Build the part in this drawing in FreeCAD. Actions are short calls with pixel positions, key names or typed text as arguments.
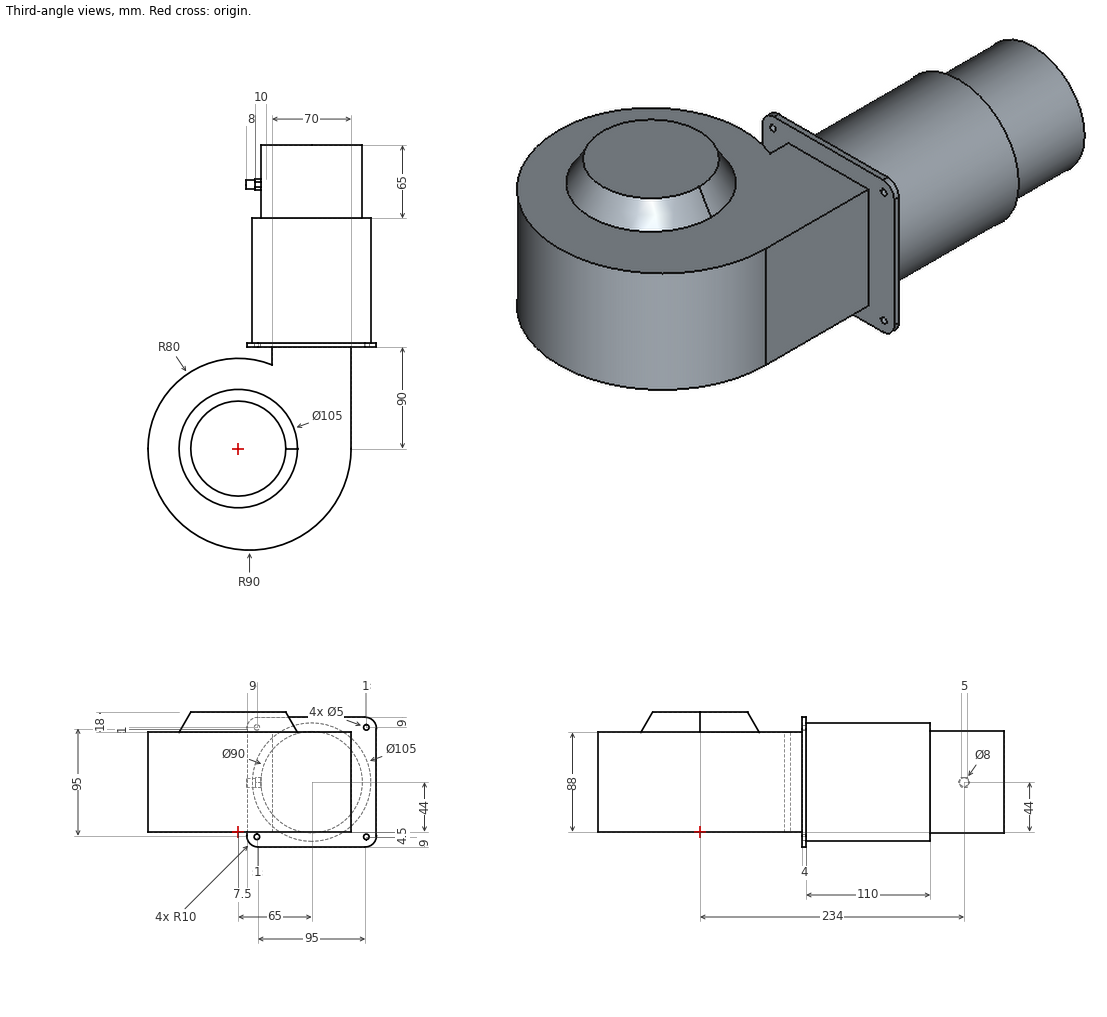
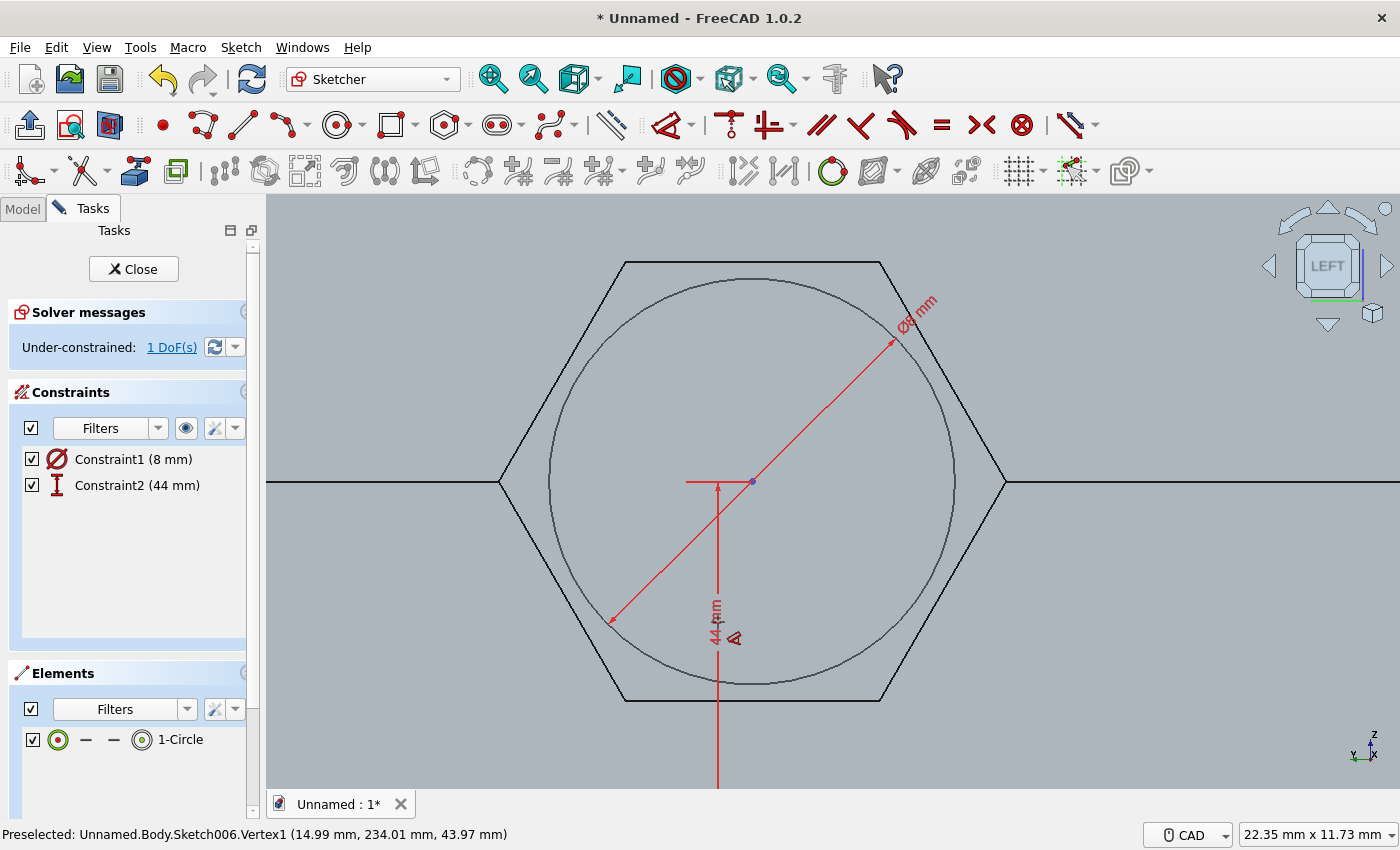
click(752, 482)
click(994, 448)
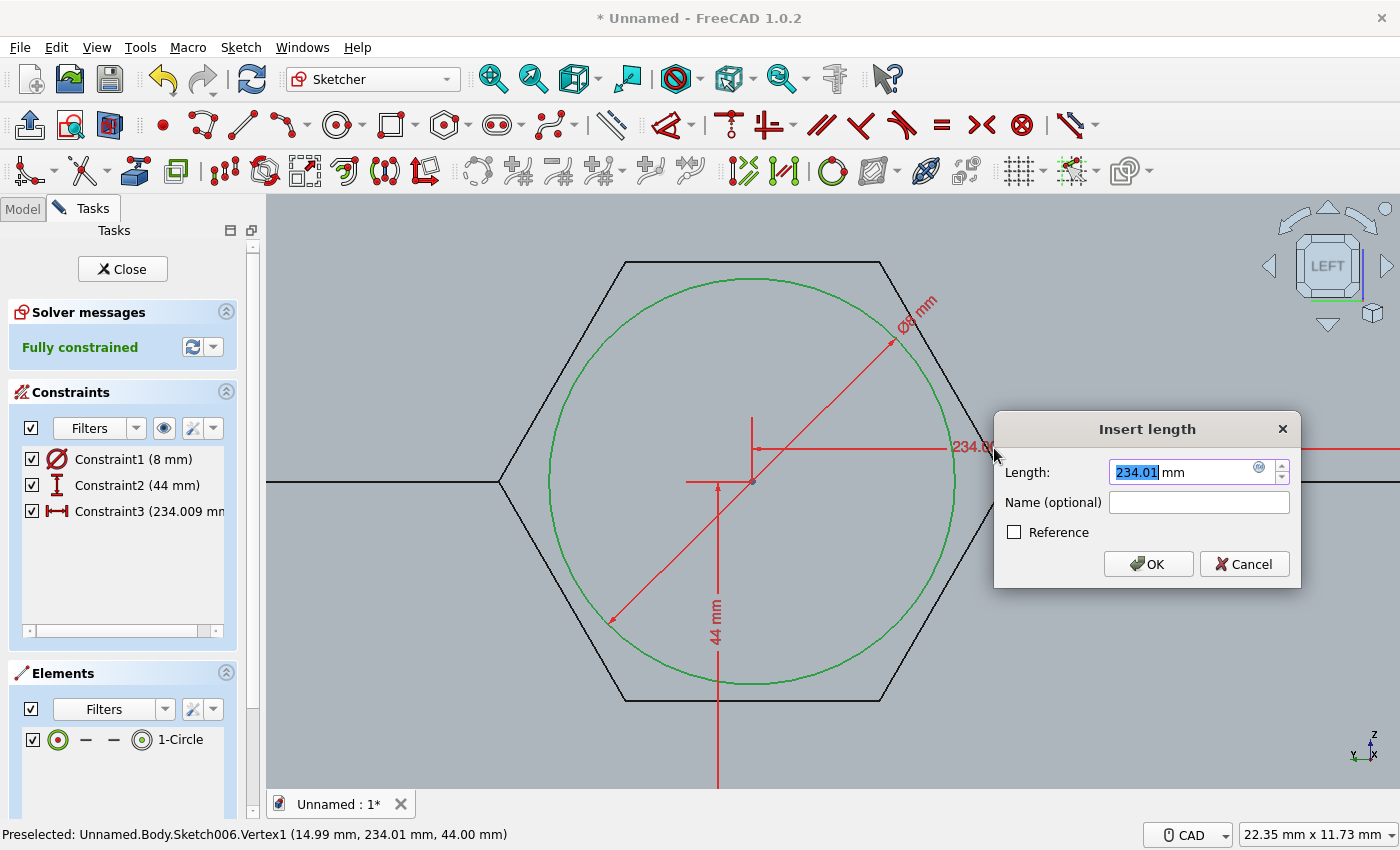
text(234)
key(Return)
key(Escape)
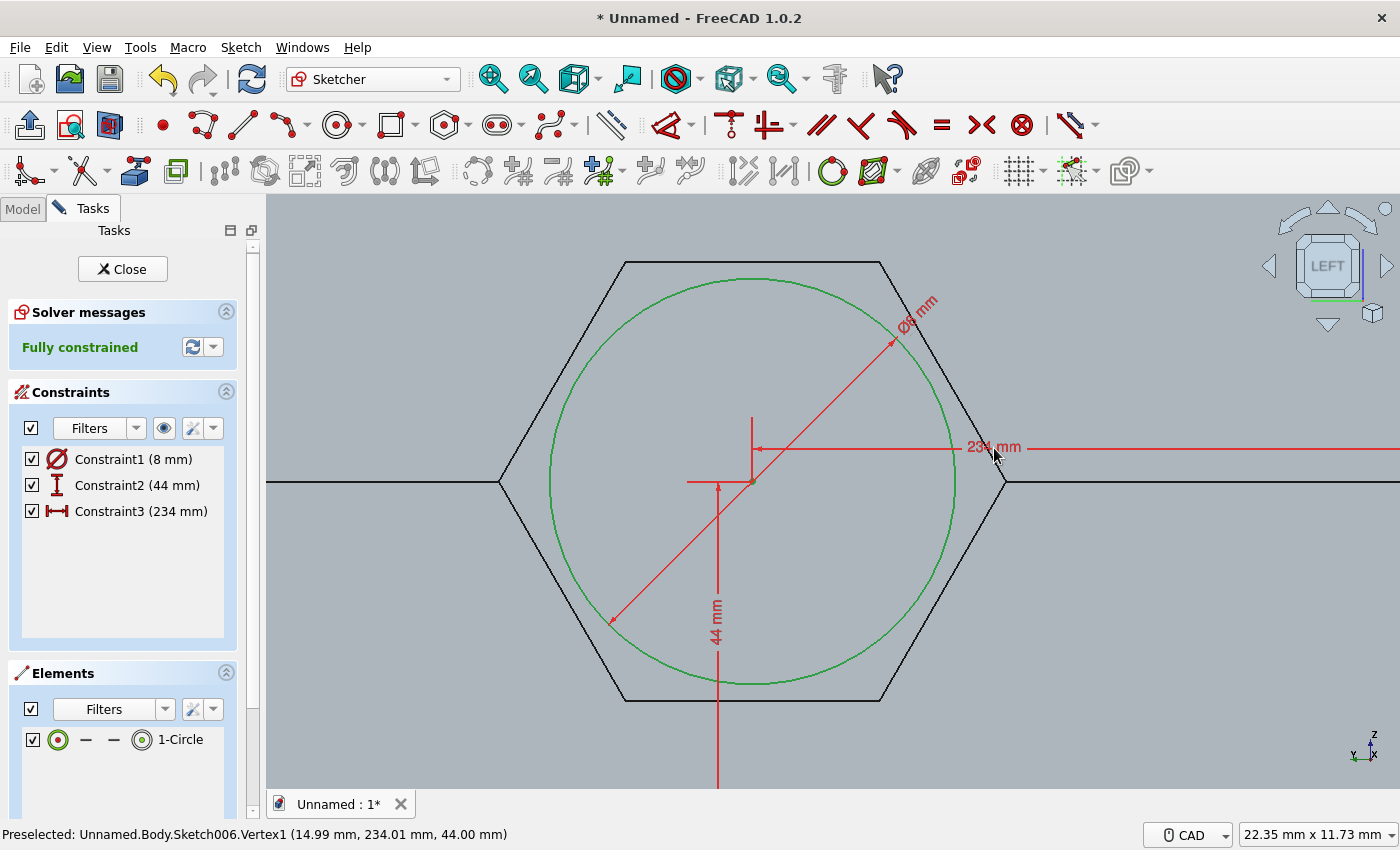
click(123, 269)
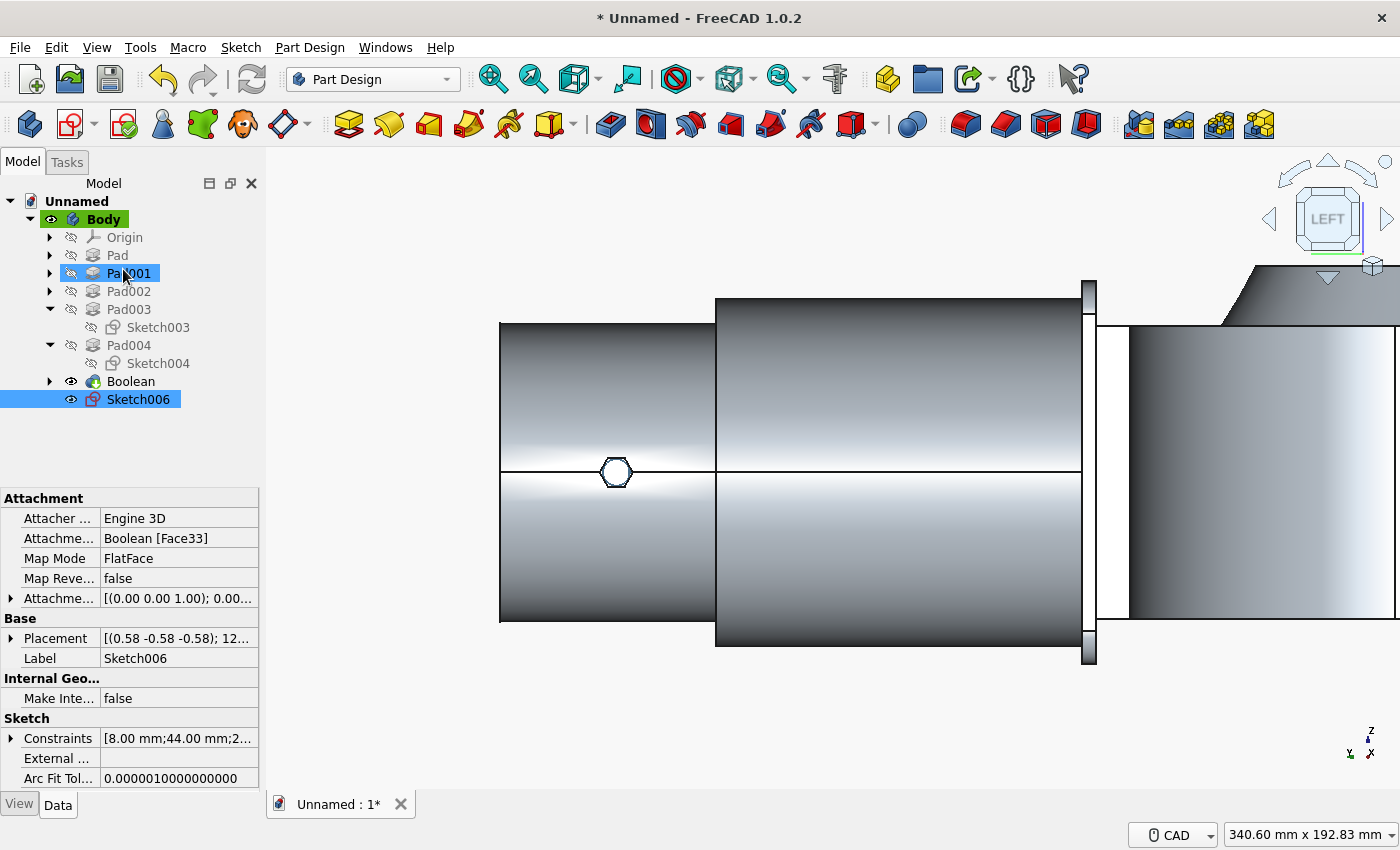
click(350, 124)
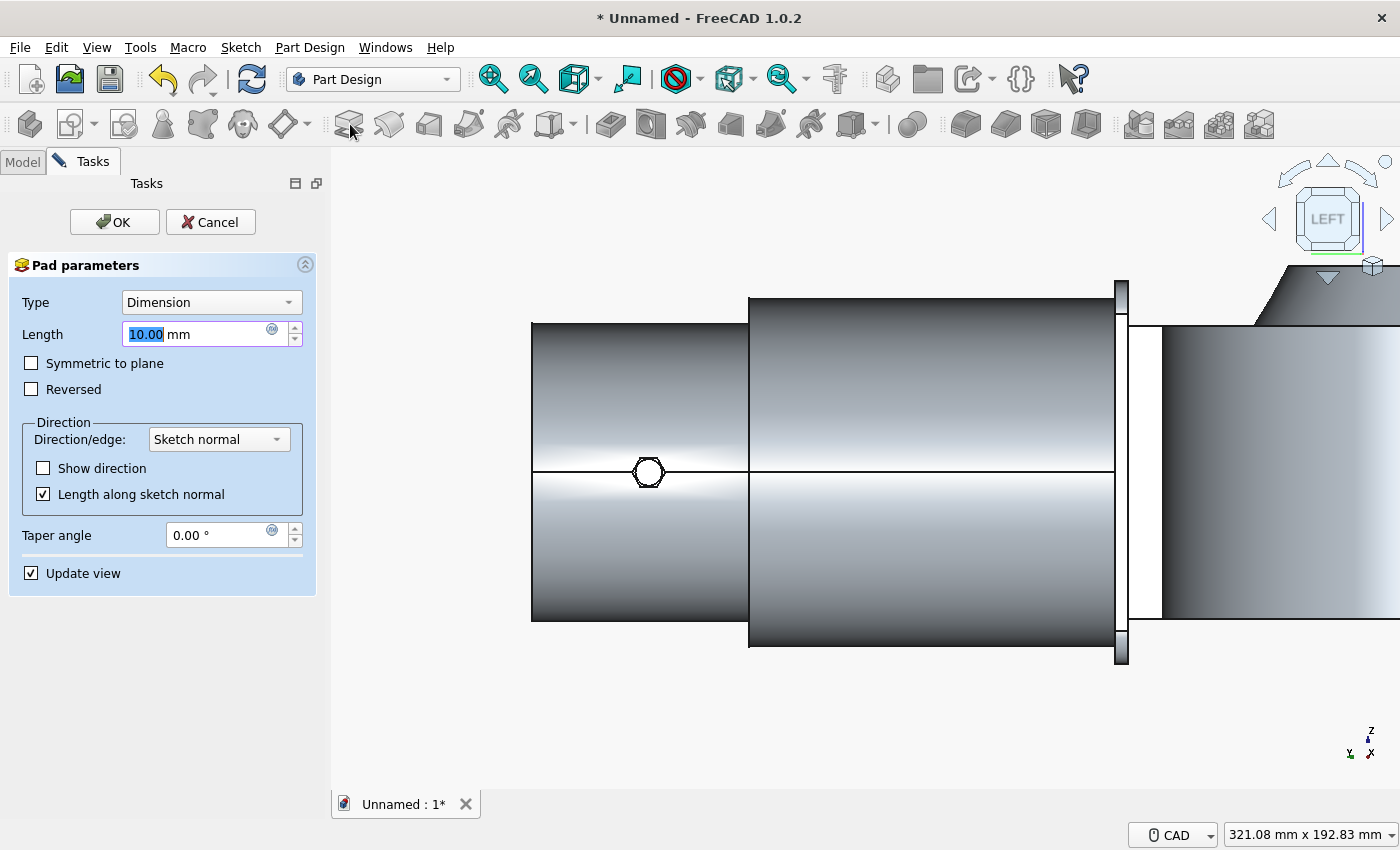
text(8)
key(Tab)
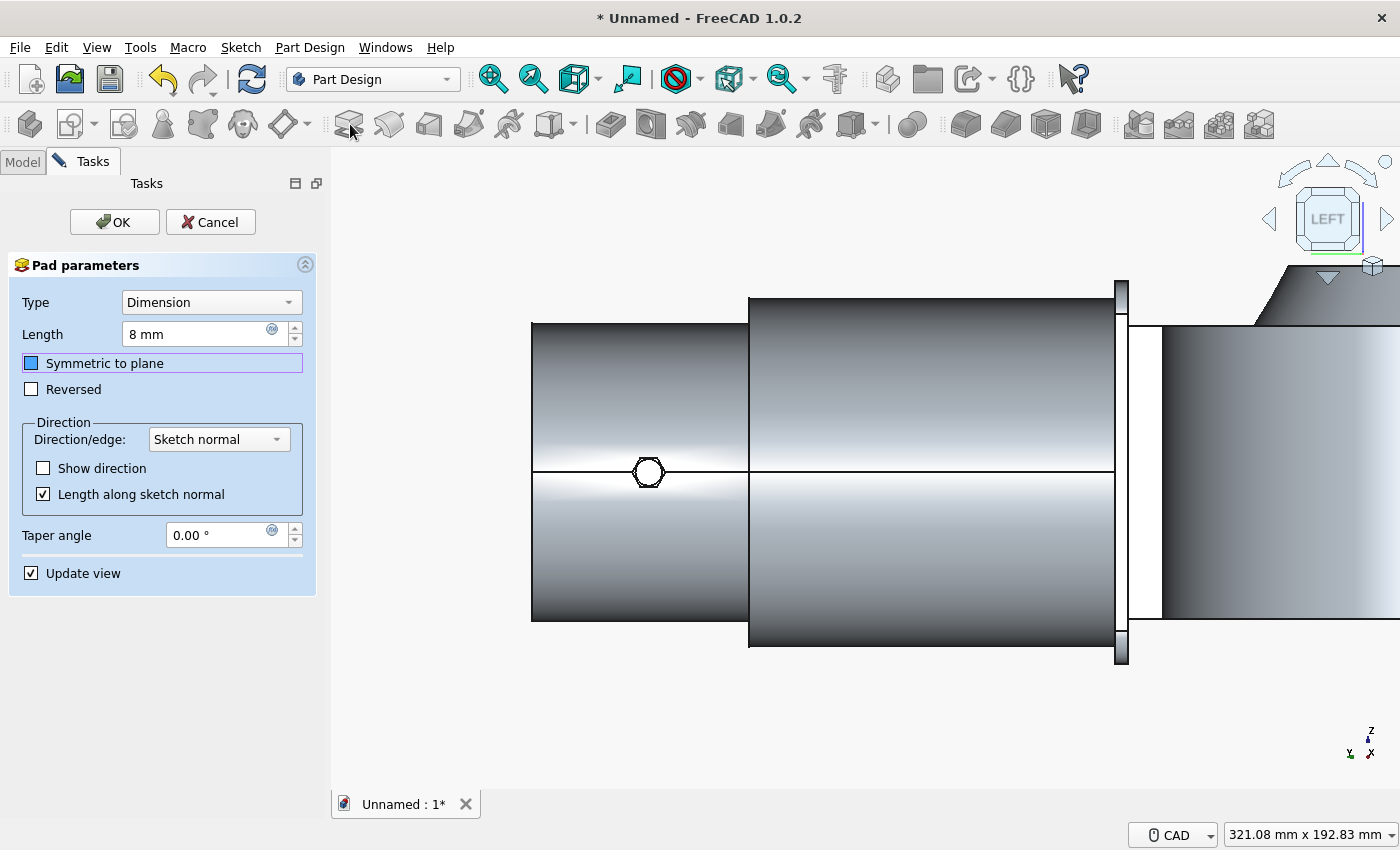
click(115, 222)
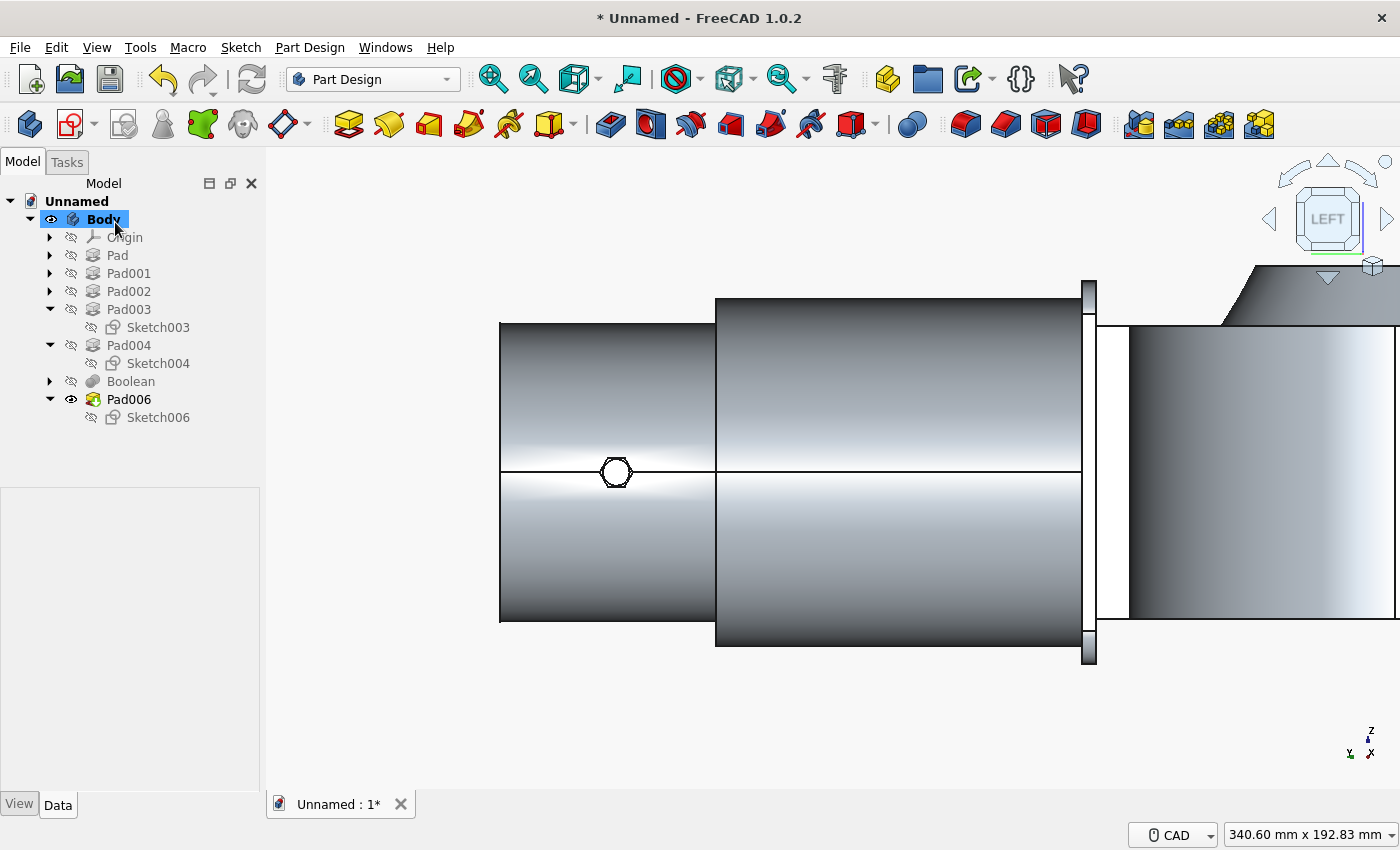
key(0)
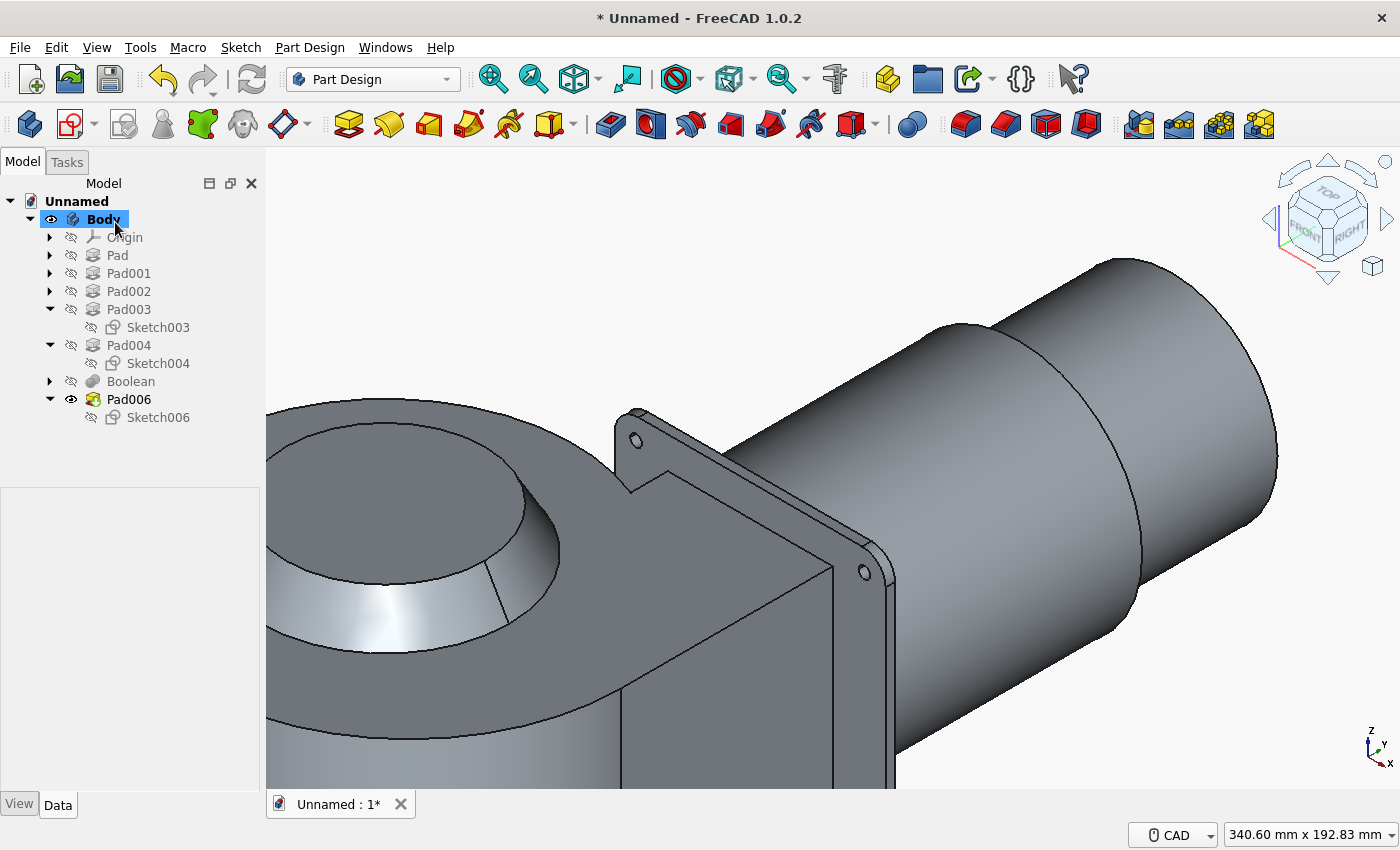
click(494, 80)